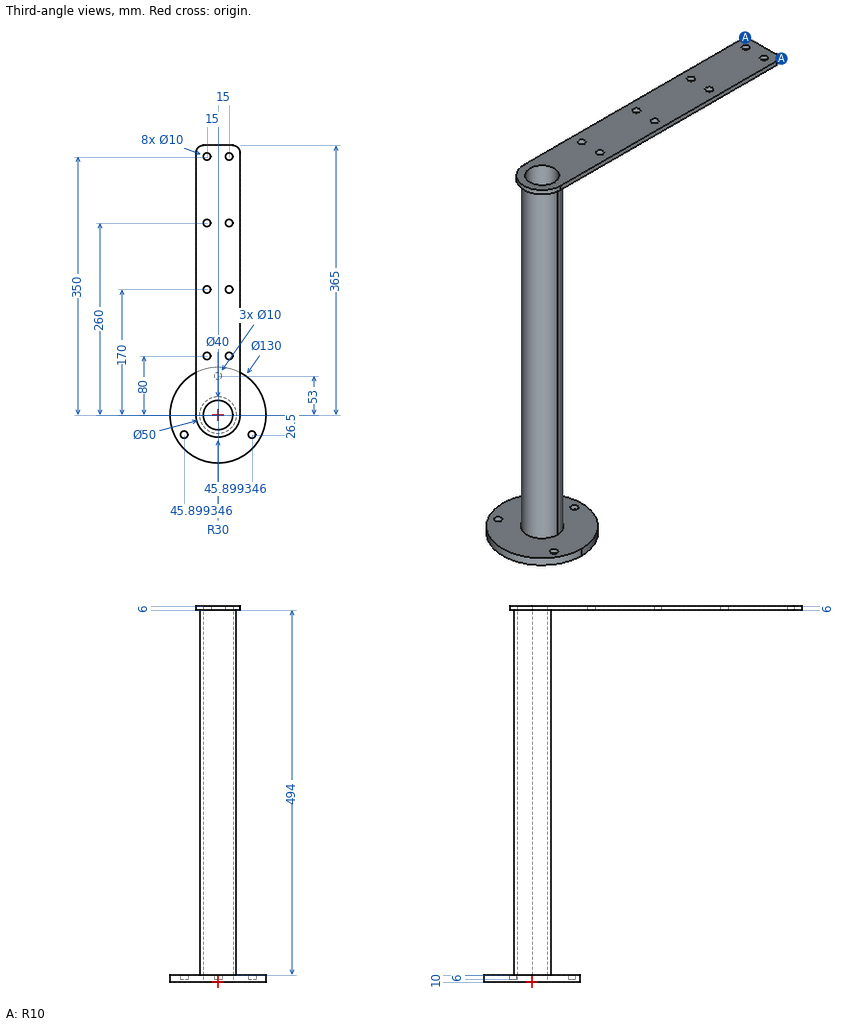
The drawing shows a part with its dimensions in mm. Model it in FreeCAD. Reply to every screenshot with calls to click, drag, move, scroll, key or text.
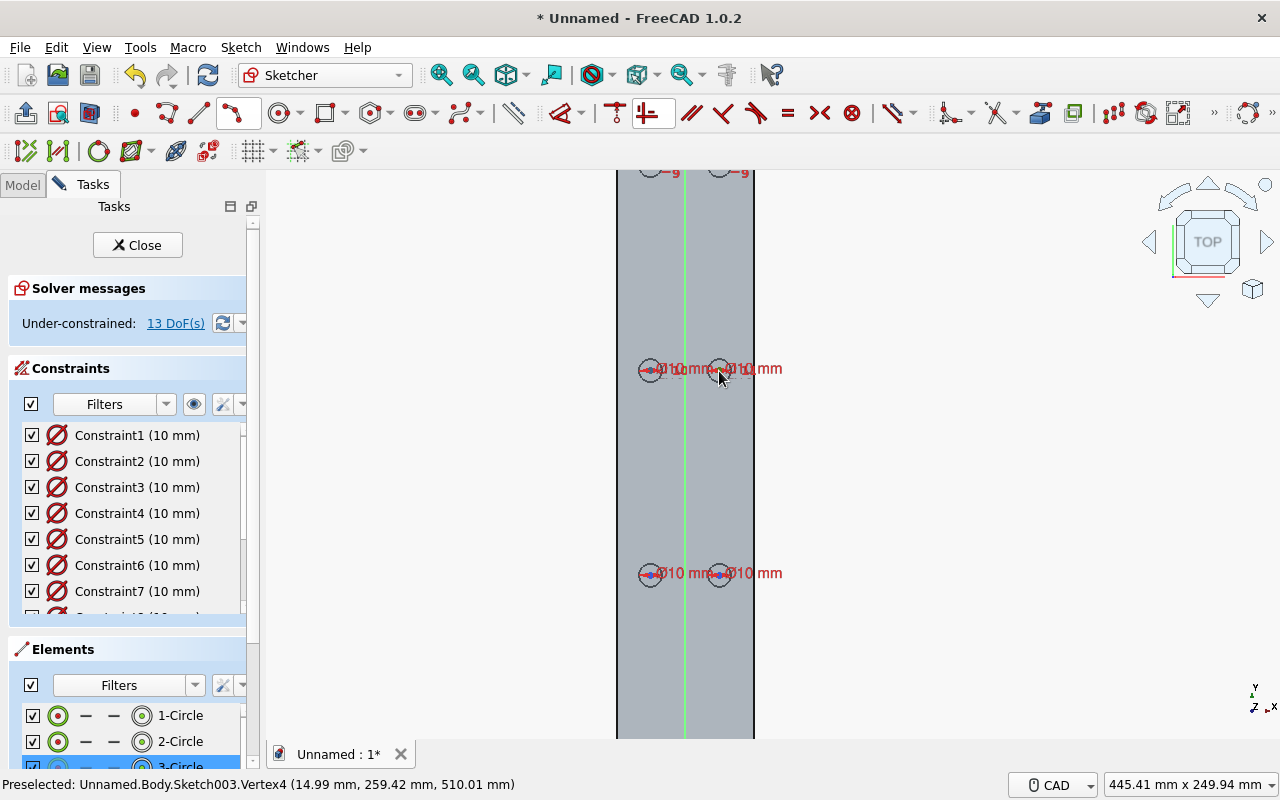
click(670, 114)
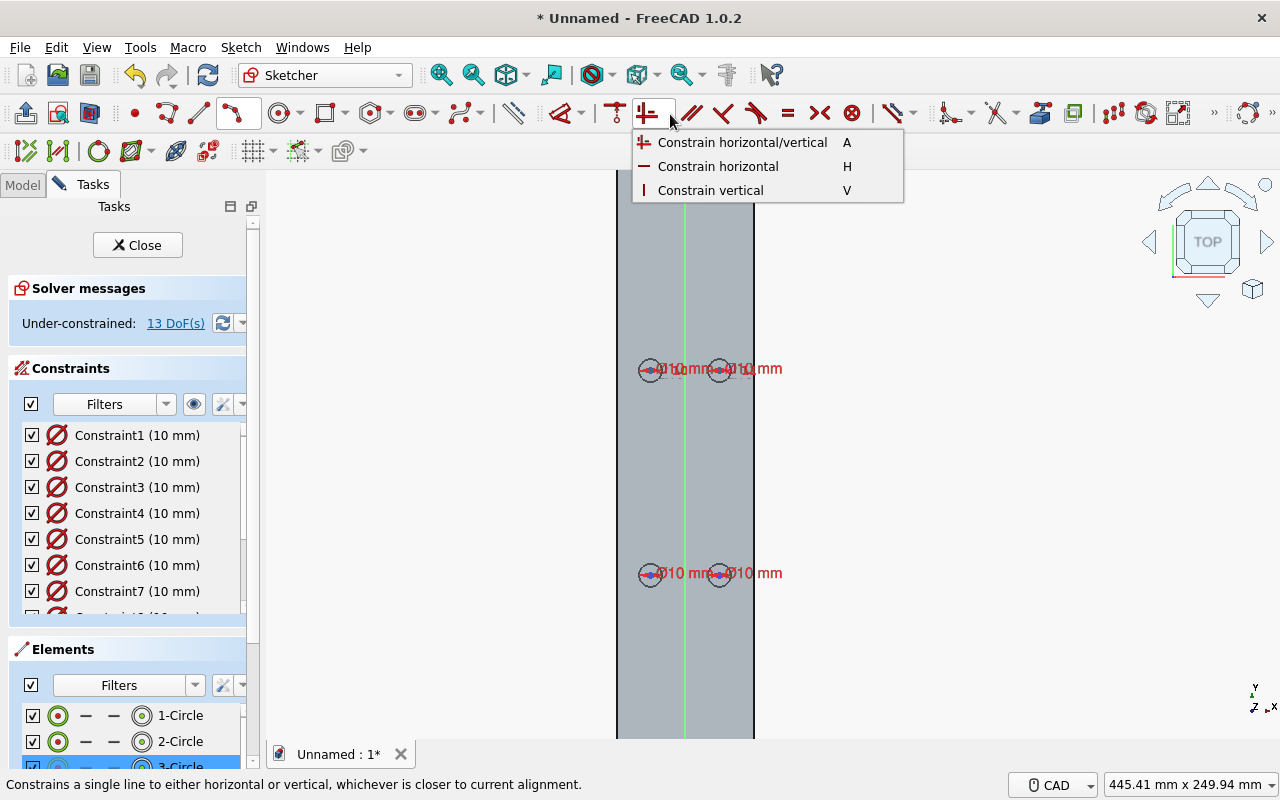
click(768, 166)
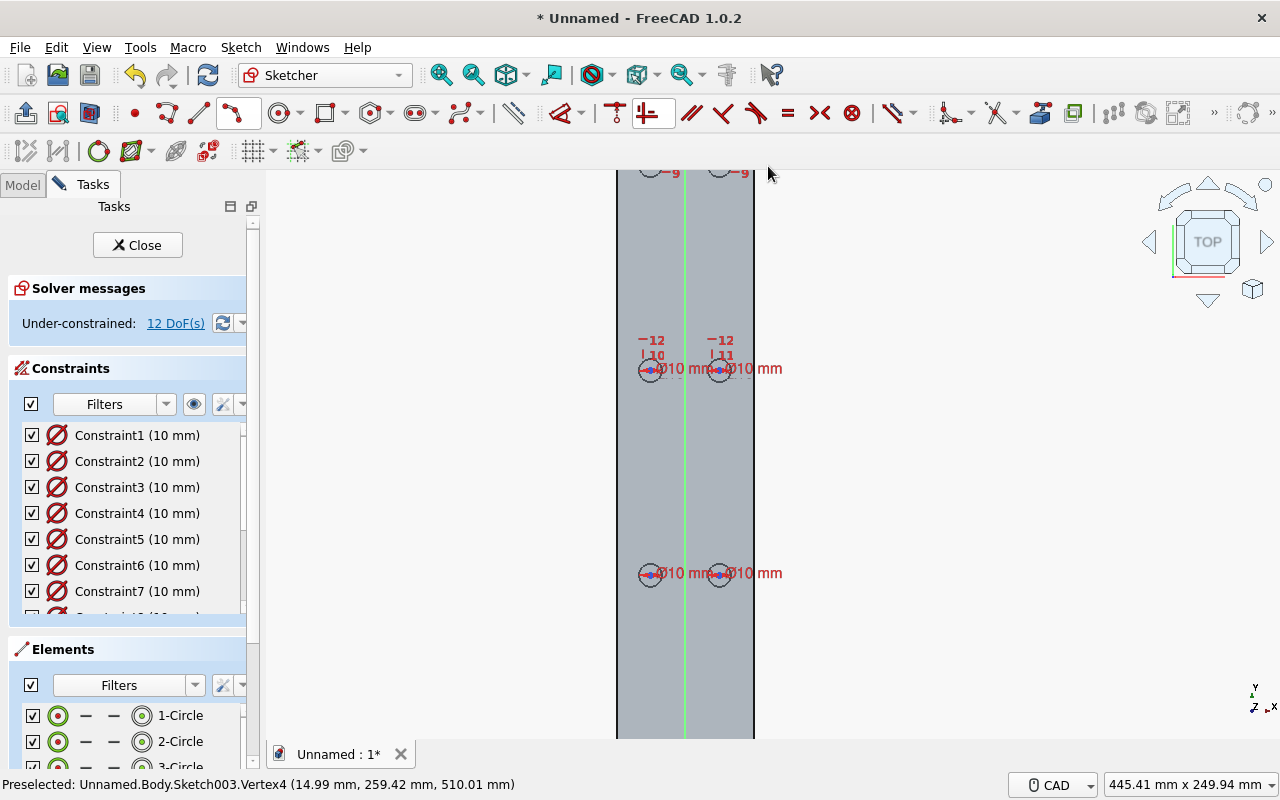
click(650, 371)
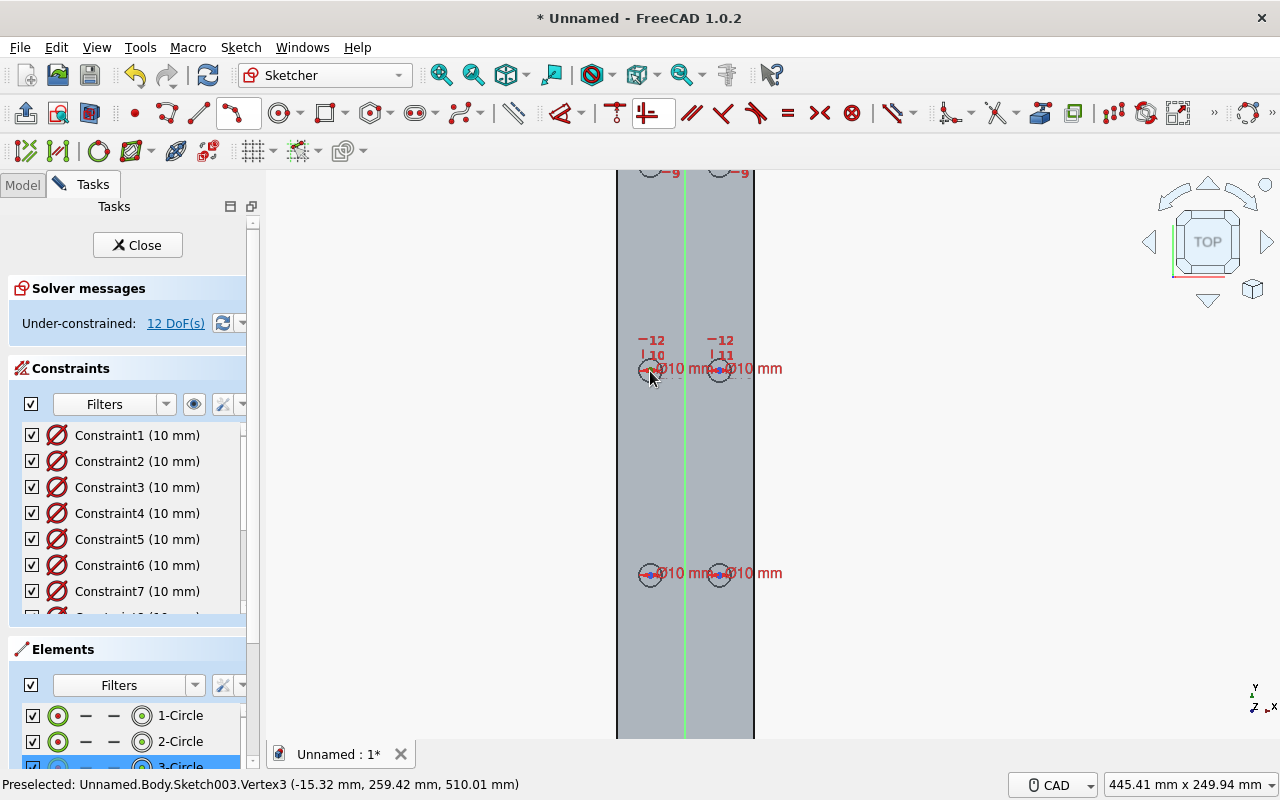
click(650, 575)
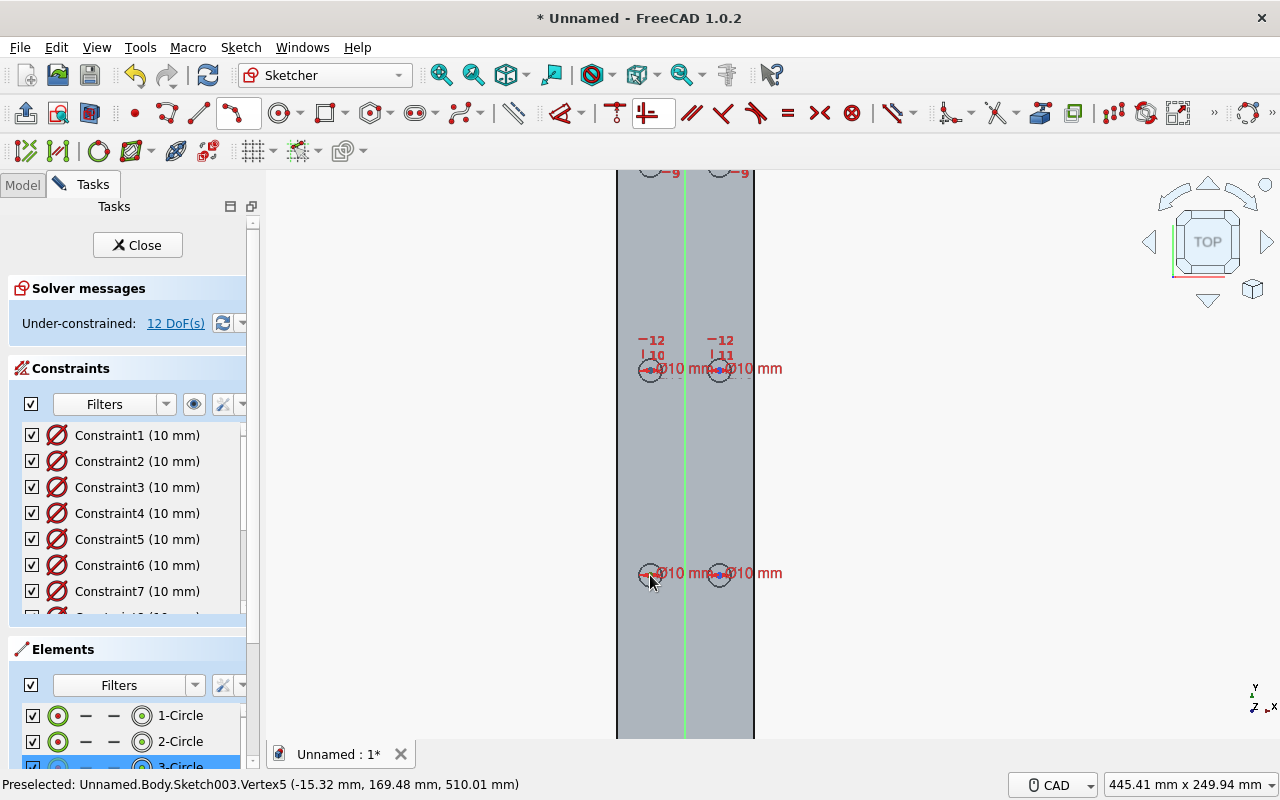
click(670, 114)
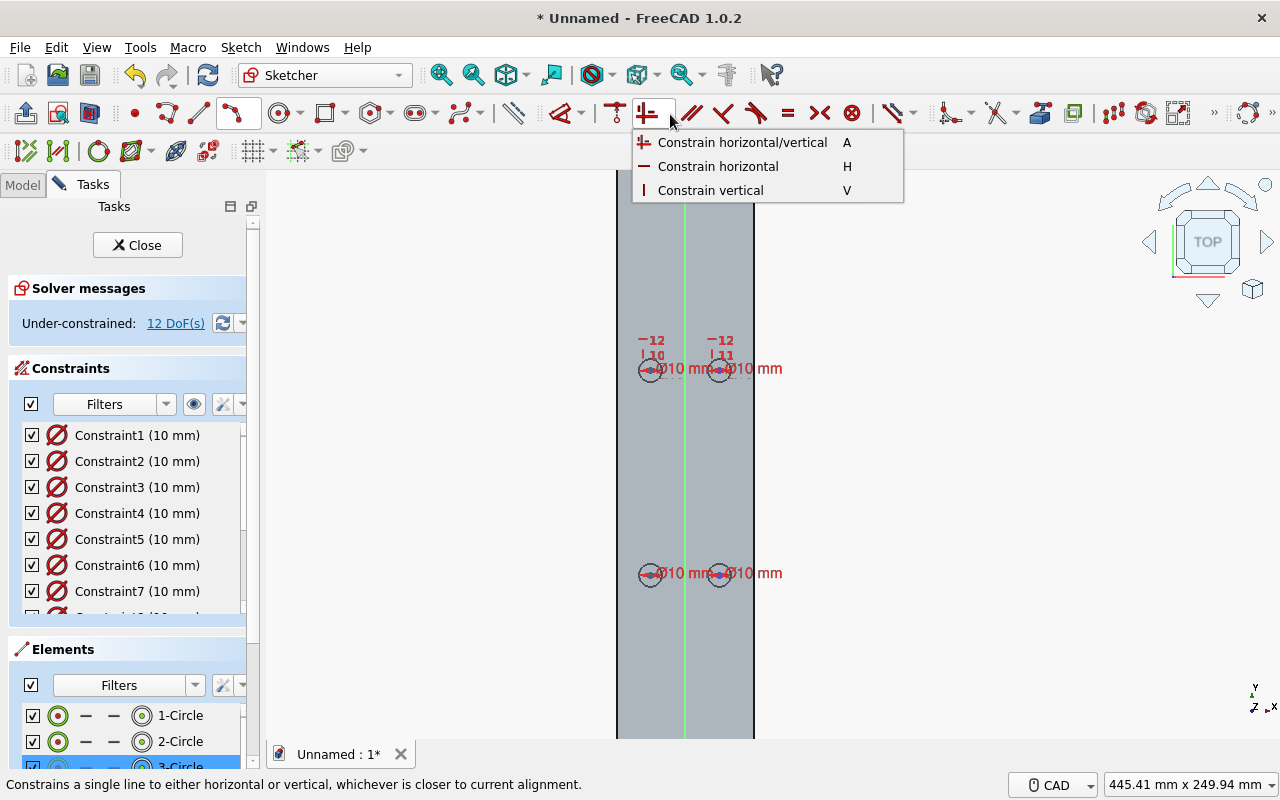
click(768, 190)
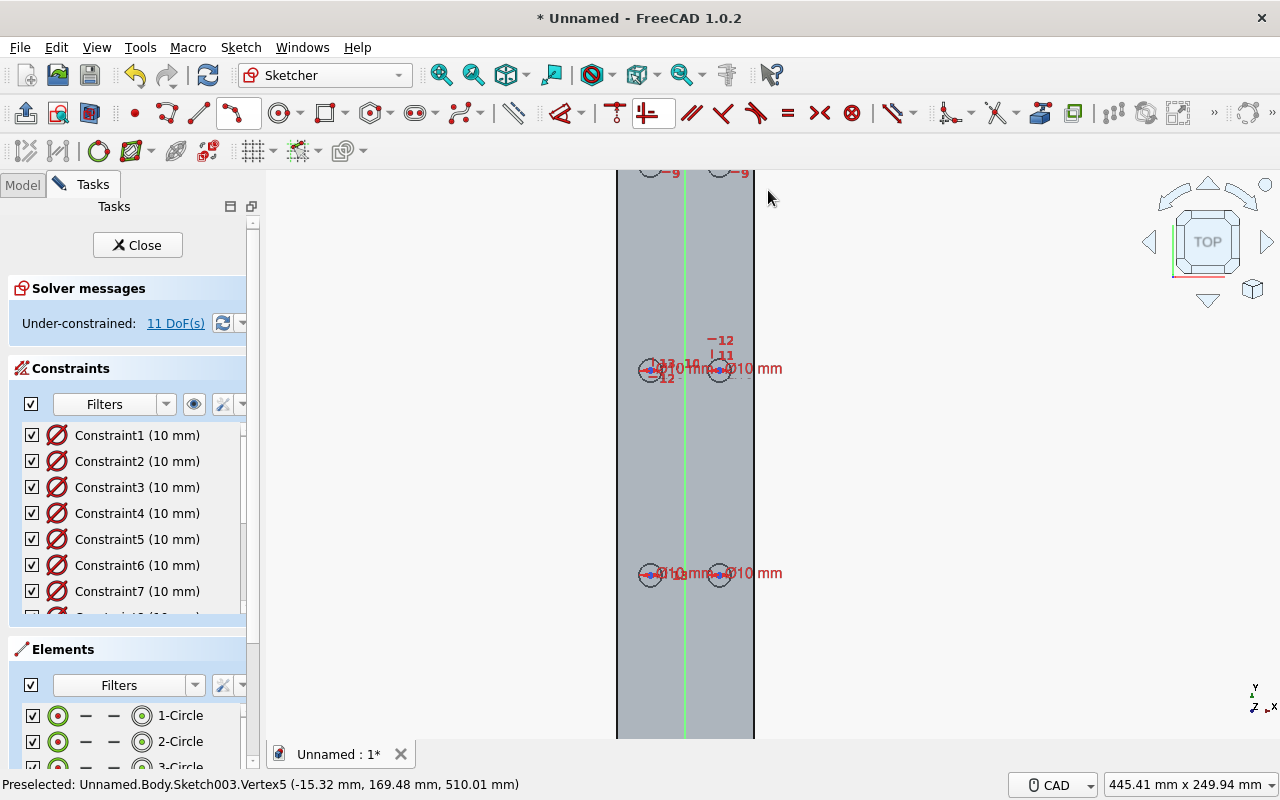
click(719, 371)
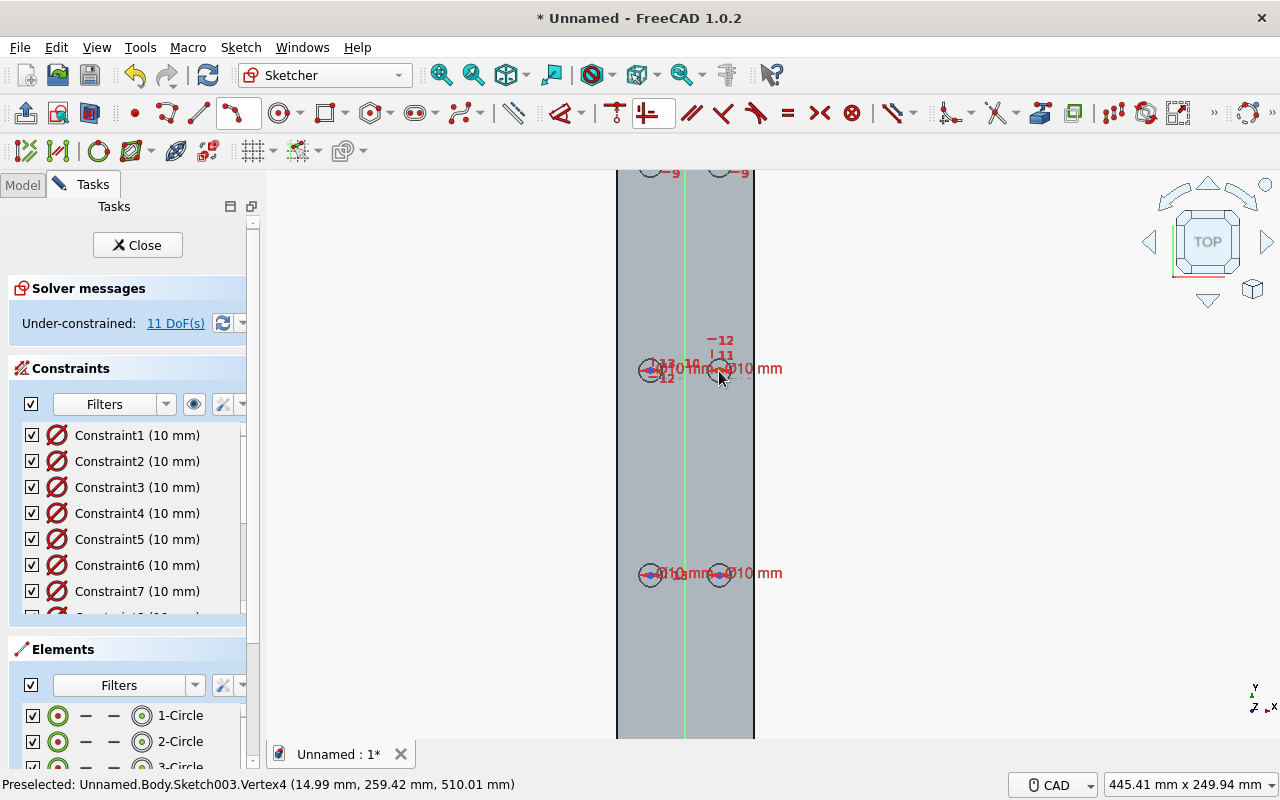
click(719, 575)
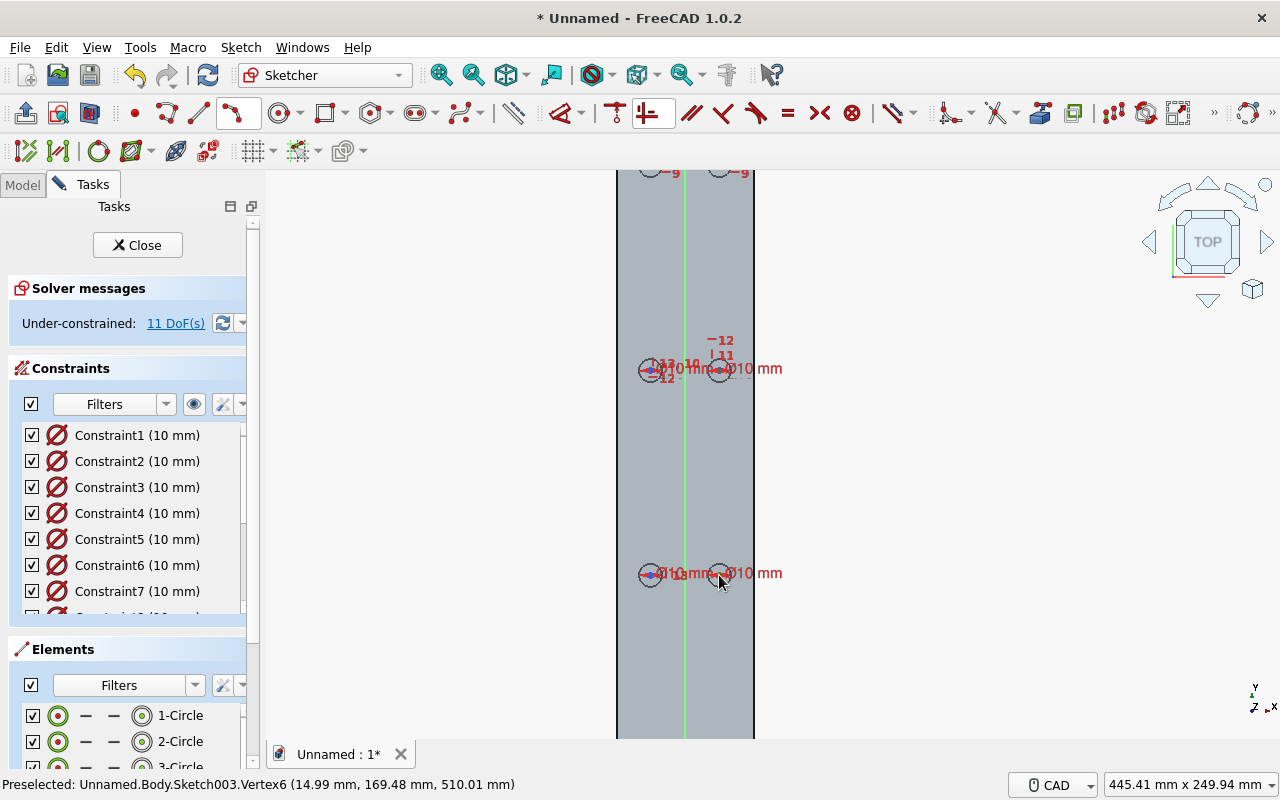
click(670, 114)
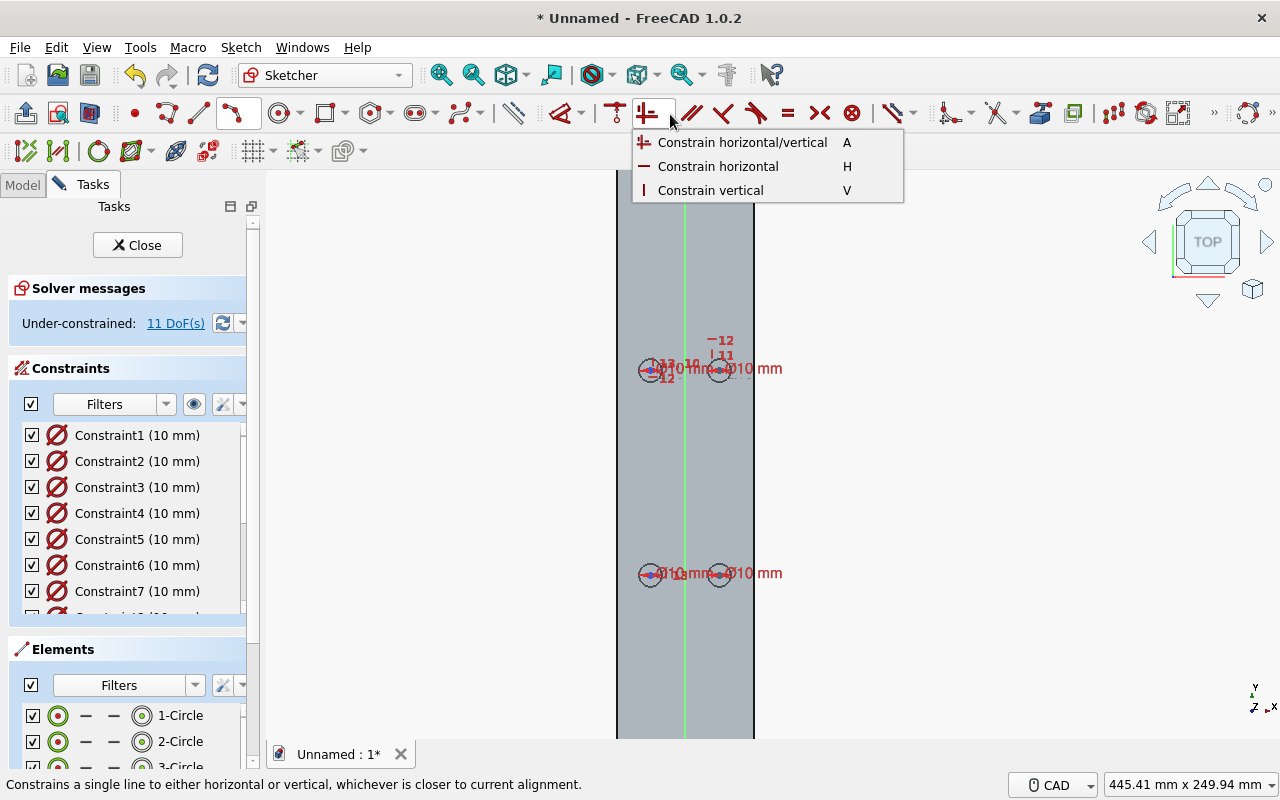
click(768, 190)